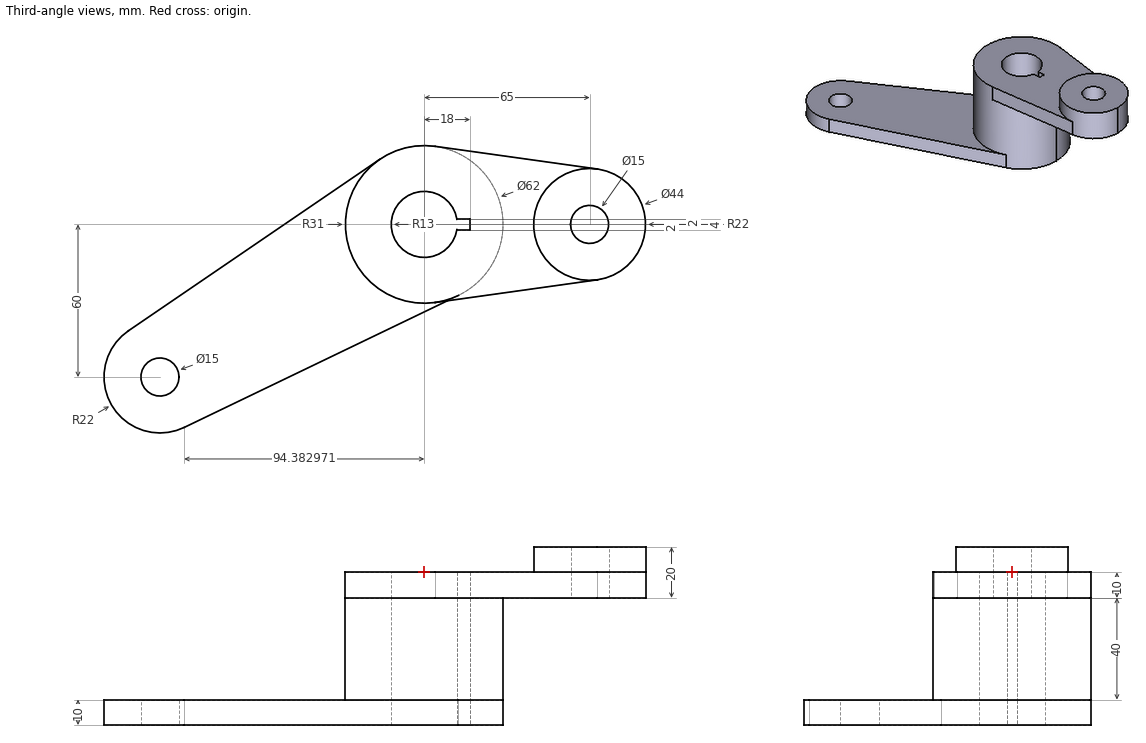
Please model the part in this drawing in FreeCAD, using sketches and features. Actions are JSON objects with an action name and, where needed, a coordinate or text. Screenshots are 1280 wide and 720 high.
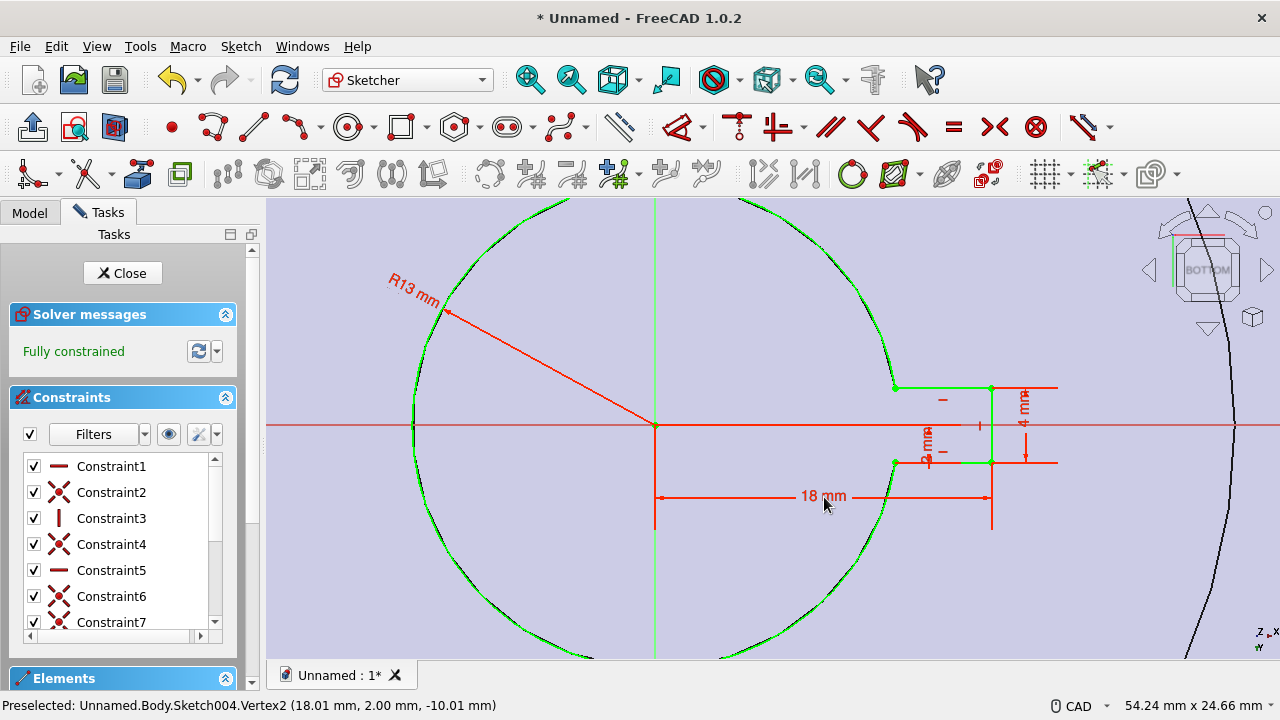
{"action": "left_click", "coordinate": [123, 273]}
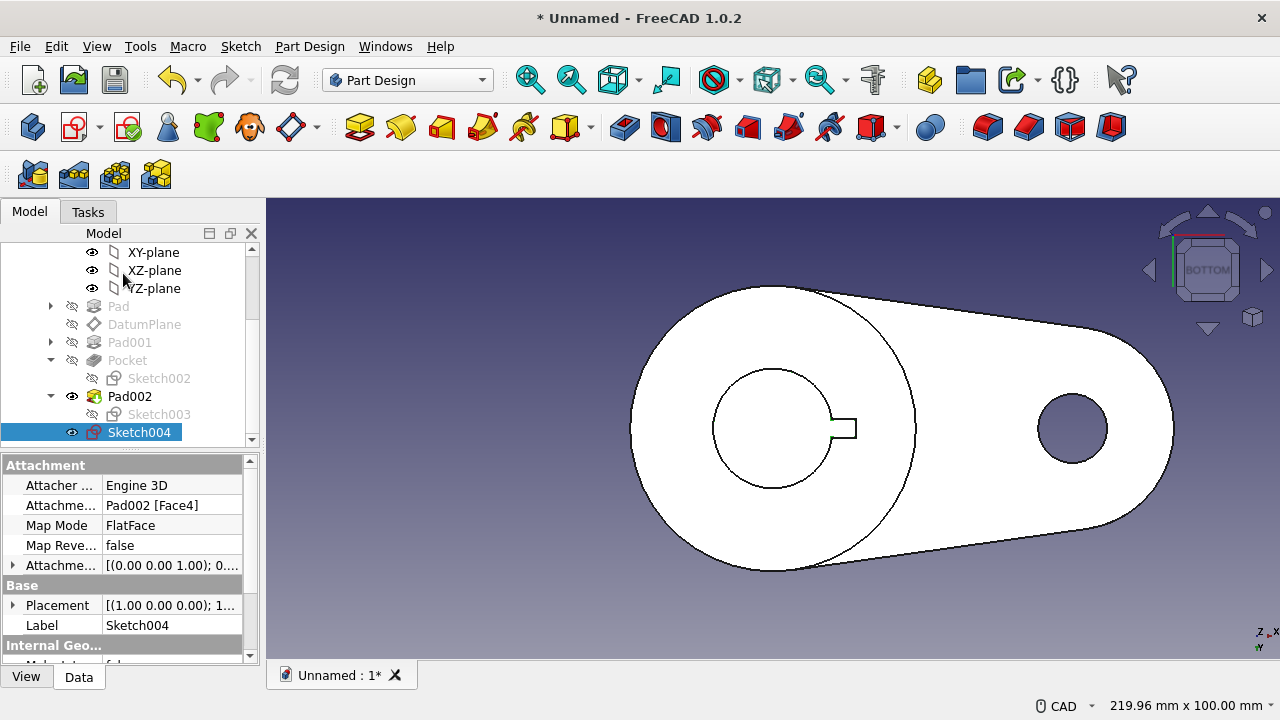
{"action": "left_click", "coordinate": [625, 128]}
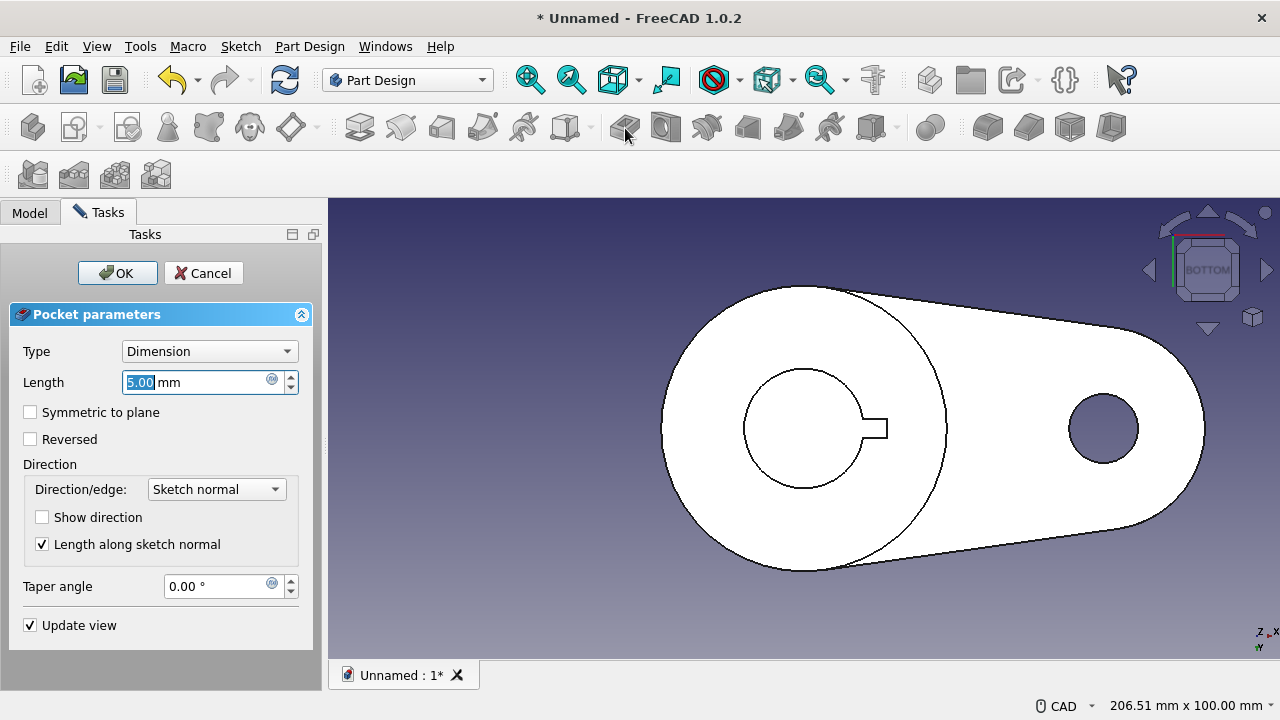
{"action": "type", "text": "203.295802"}
{"action": "key", "text": "Tab"}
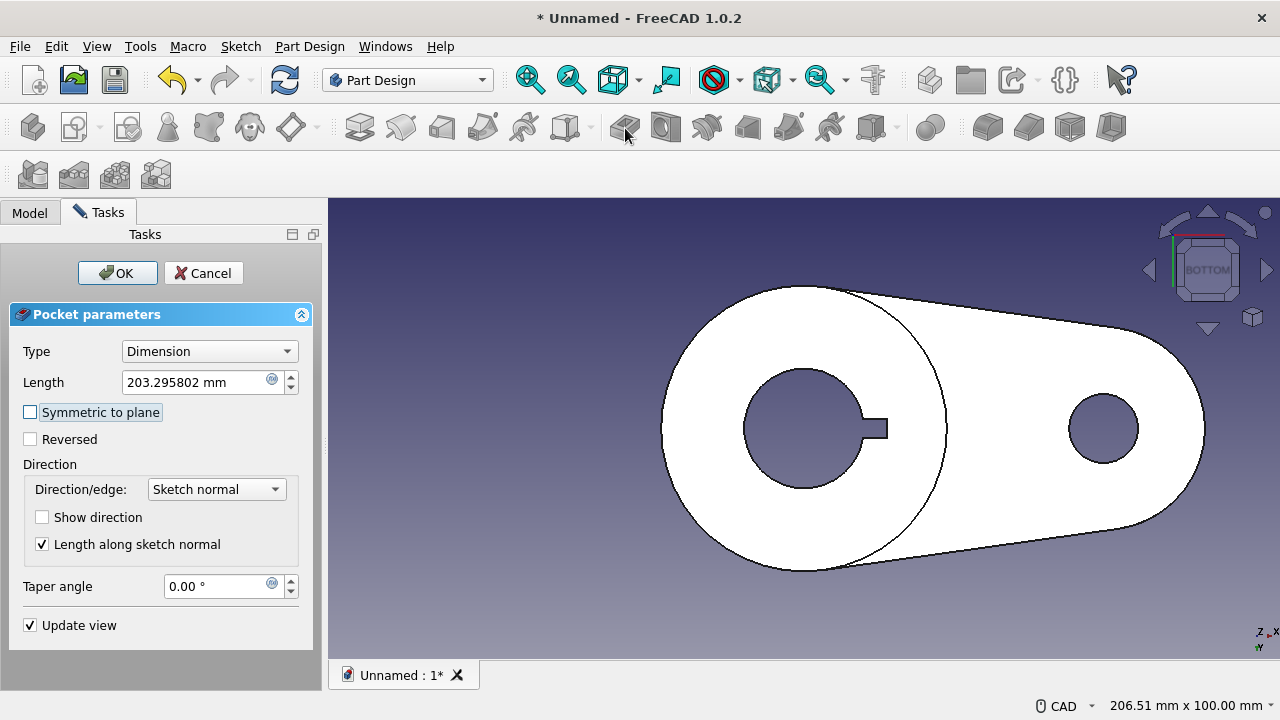
{"action": "left_click", "coordinate": [31, 412]}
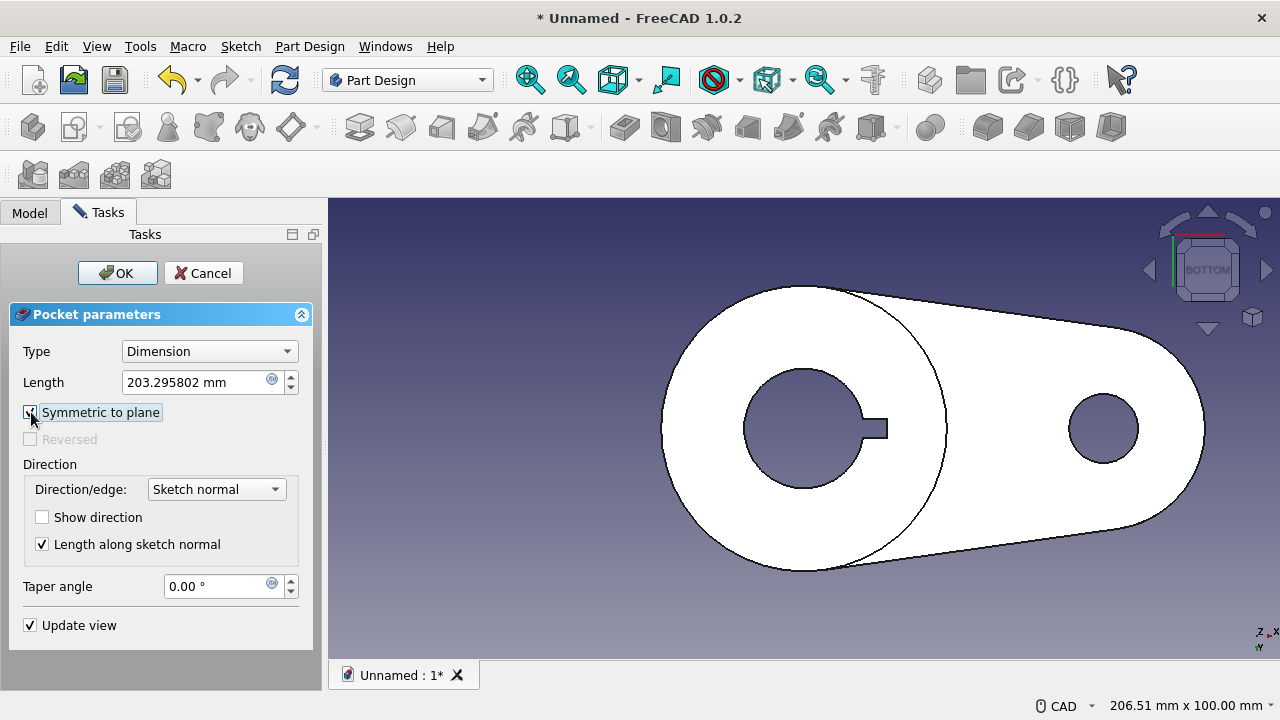
{"action": "left_click", "coordinate": [118, 273]}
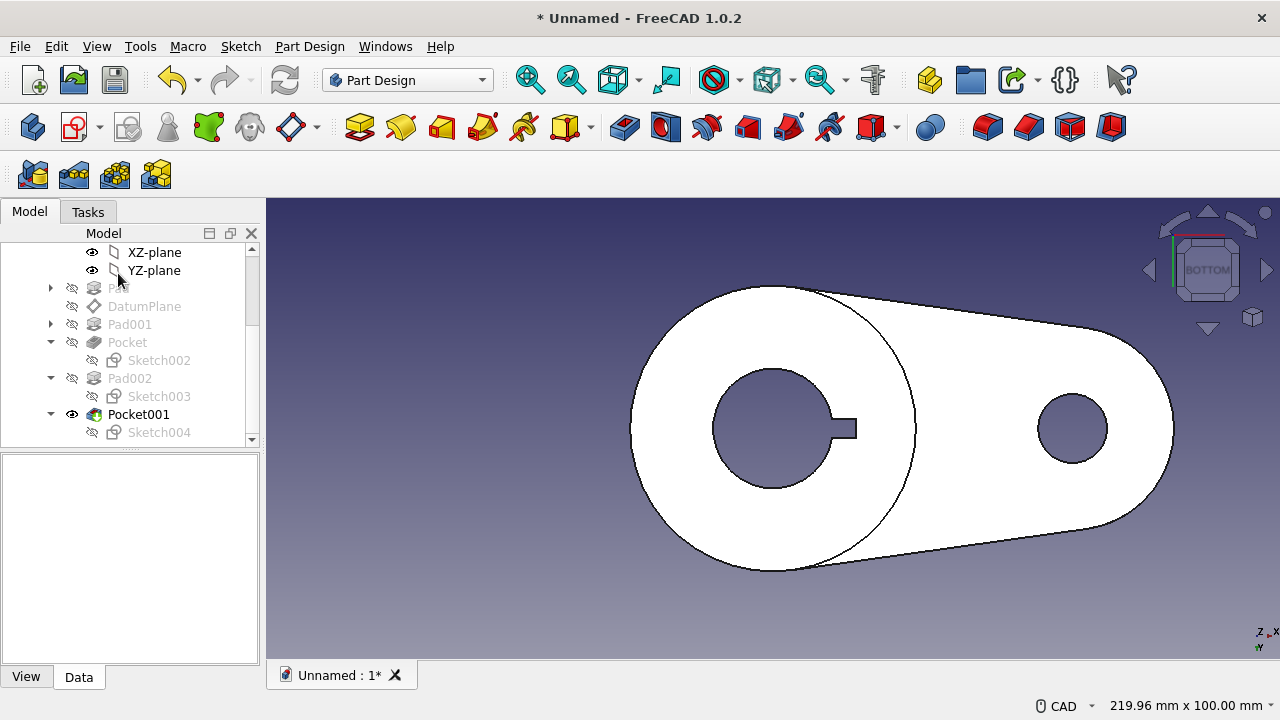
{"action": "left_click", "coordinate": [855, 387]}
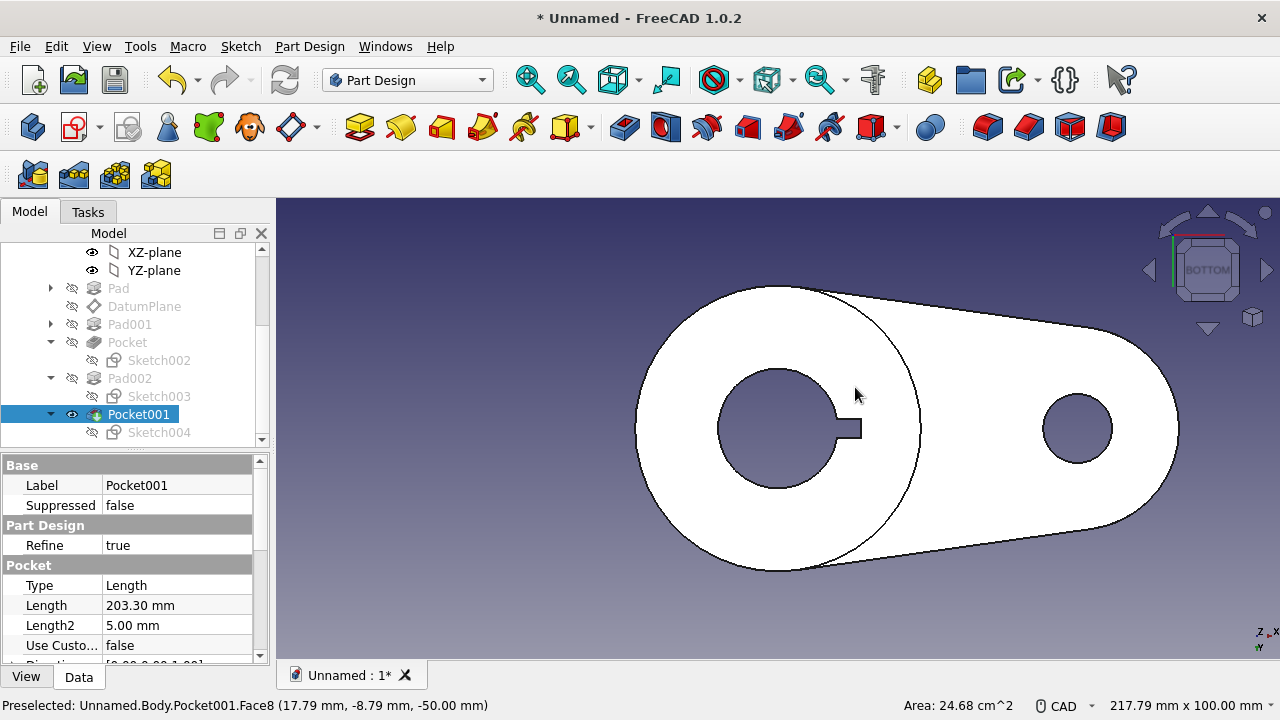
{"action": "left_click", "coordinate": [74, 128]}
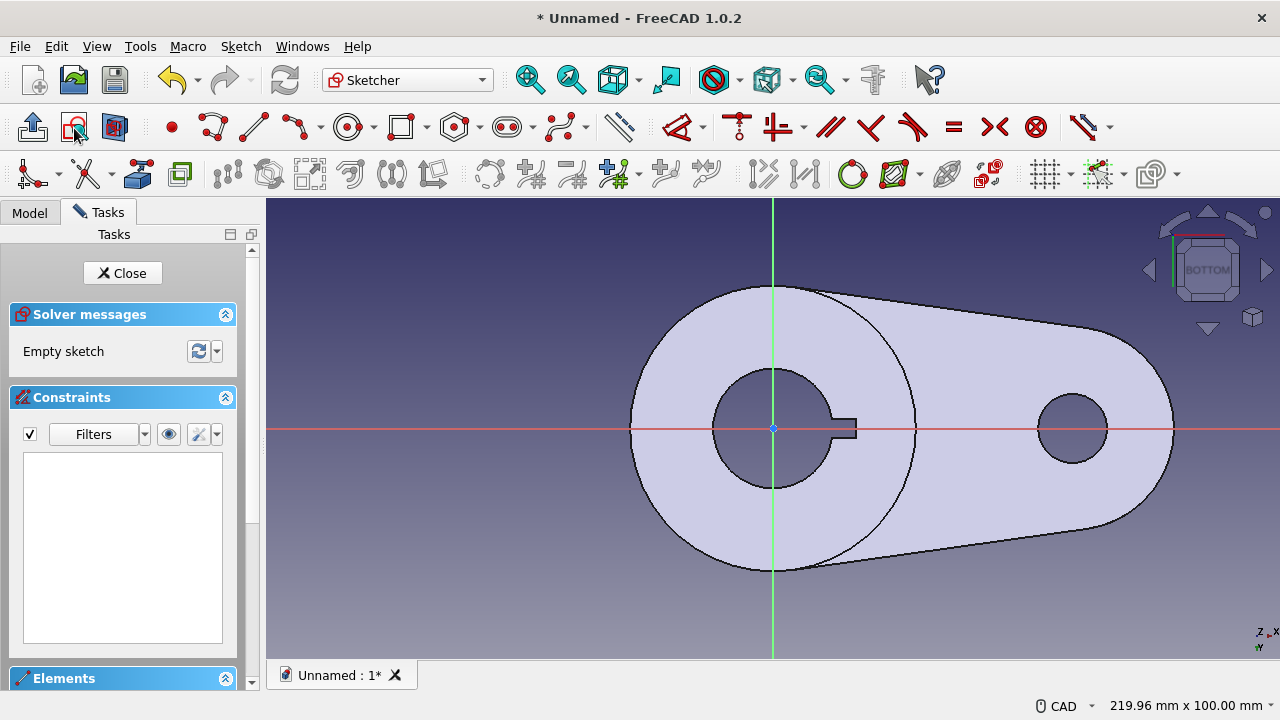
{"action": "scroll", "coordinate": [891, 581], "scroll_direction": "down", "scroll_amount": 3}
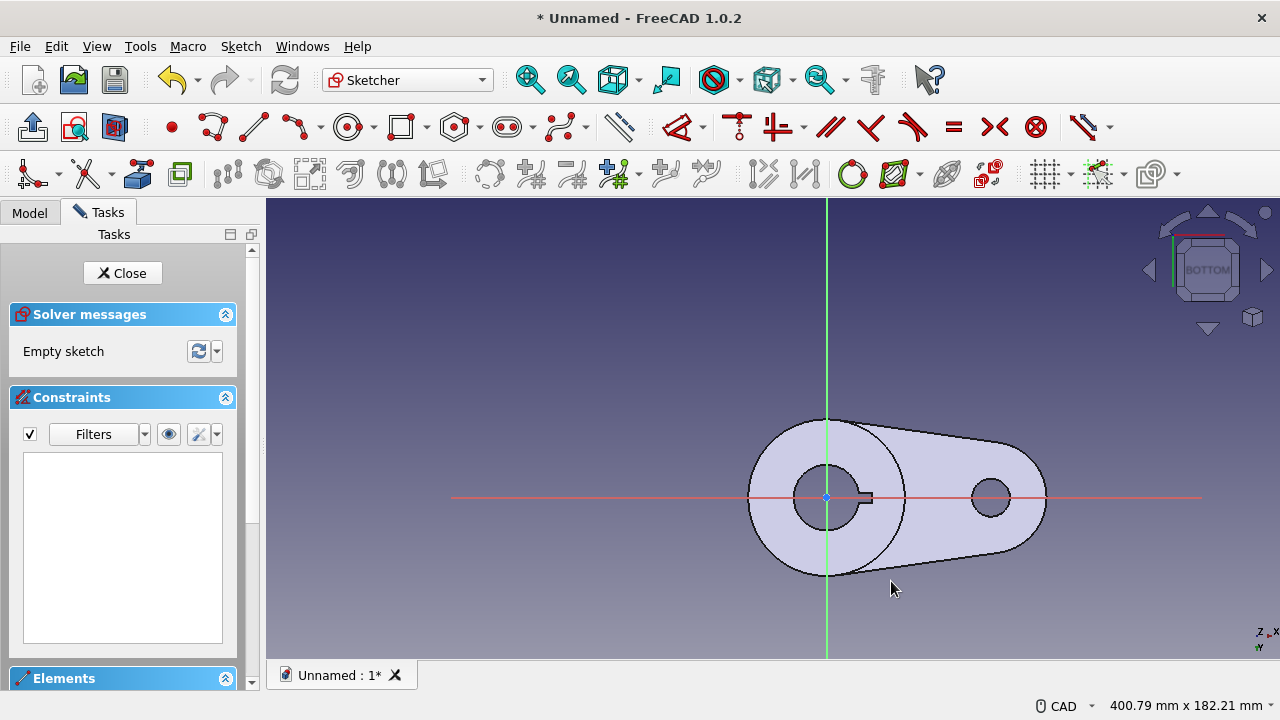
{"action": "key", "text": "g l"}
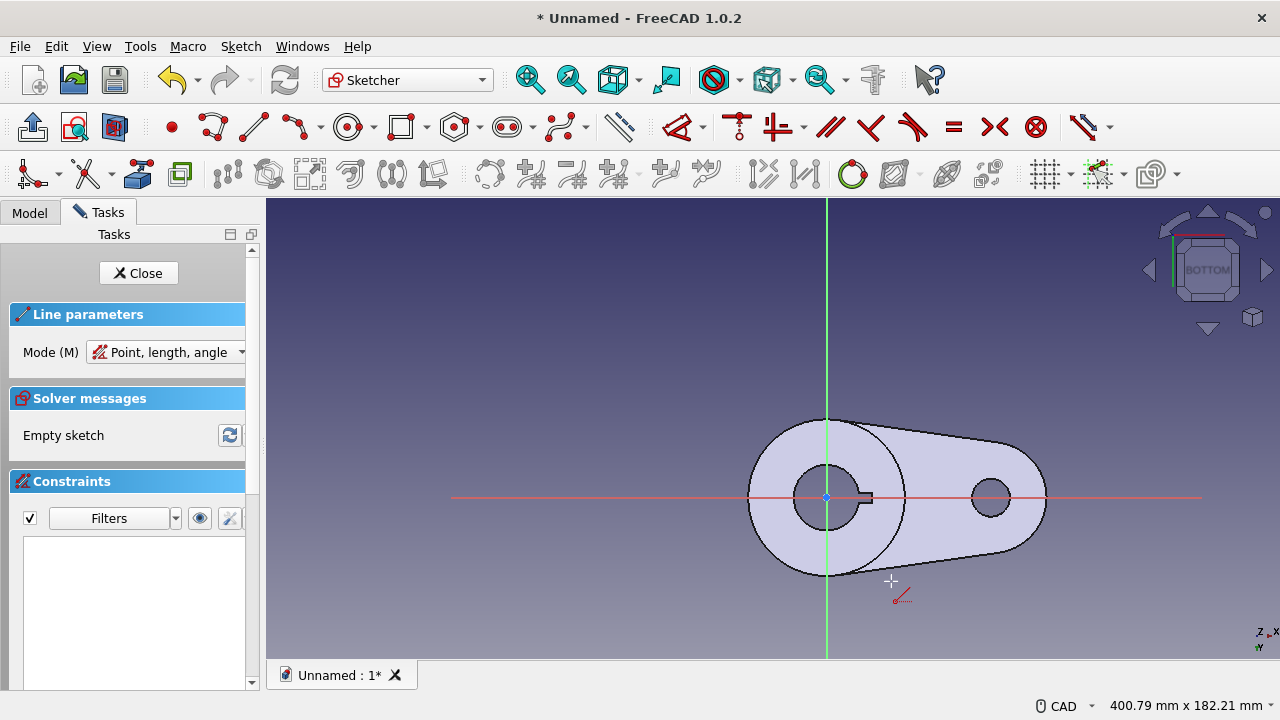
{"action": "left_click", "coordinate": [782, 562]}
{"action": "left_click", "coordinate": [532, 392]}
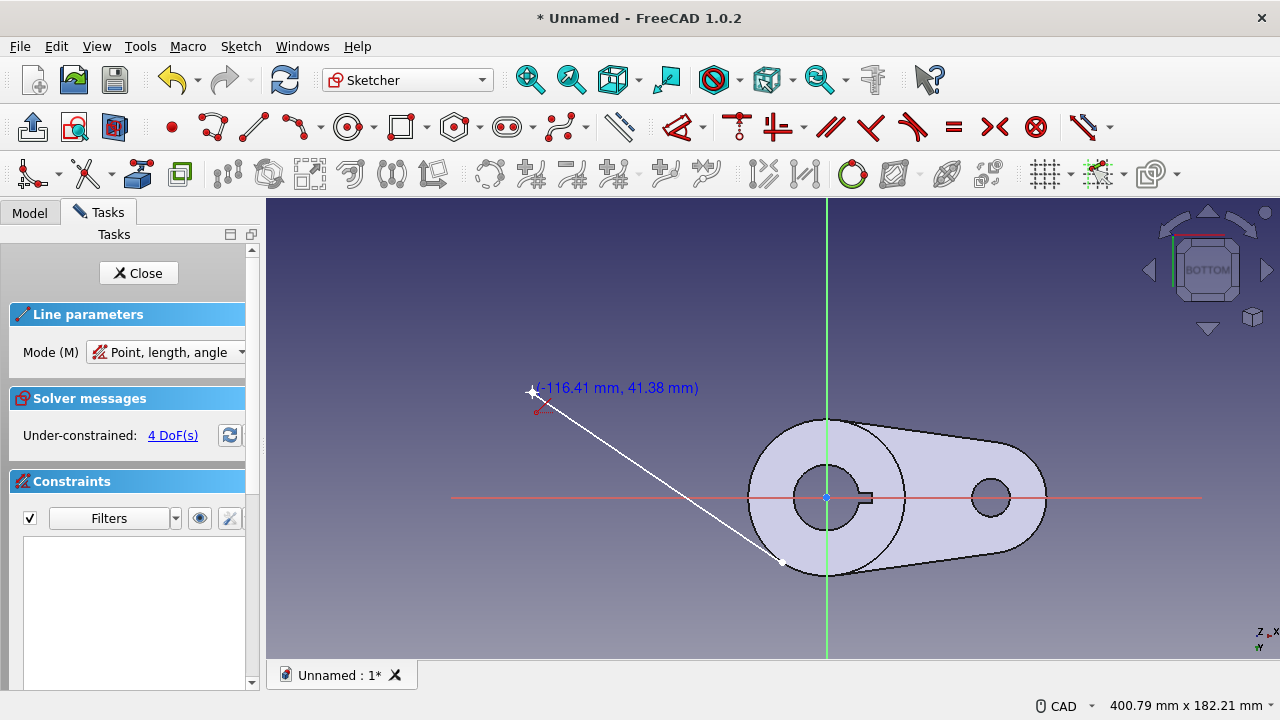
{"action": "left_click", "coordinate": [588, 296]}
{"action": "left_click", "coordinate": [861, 427]}